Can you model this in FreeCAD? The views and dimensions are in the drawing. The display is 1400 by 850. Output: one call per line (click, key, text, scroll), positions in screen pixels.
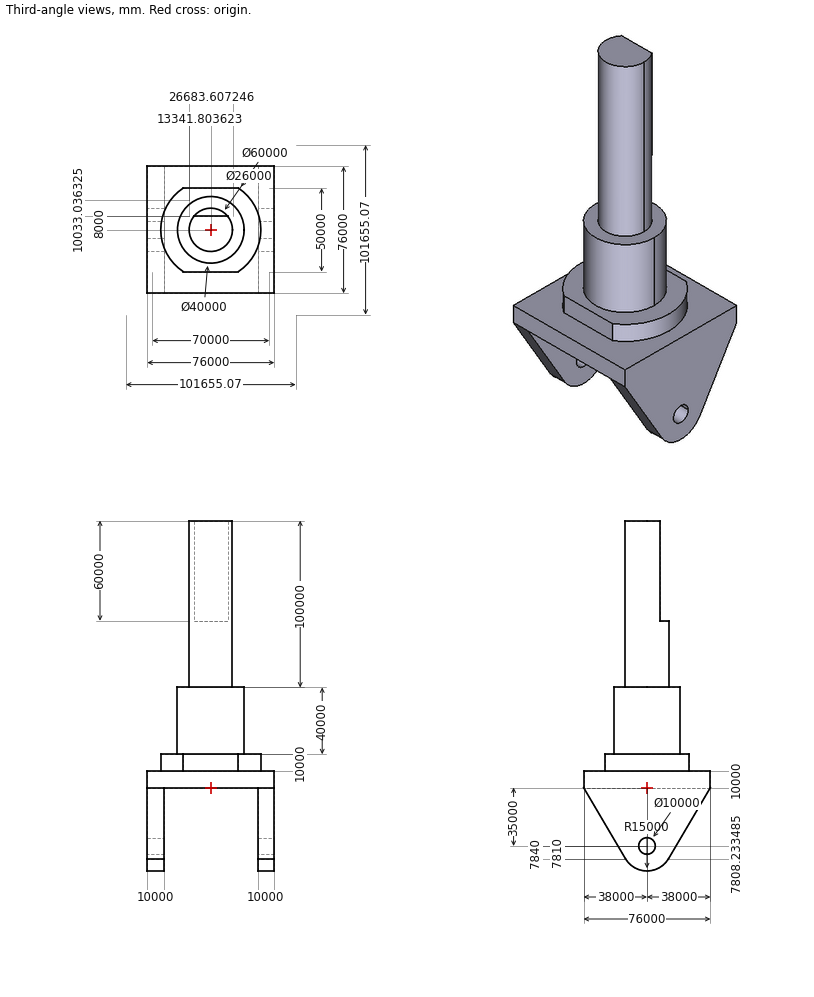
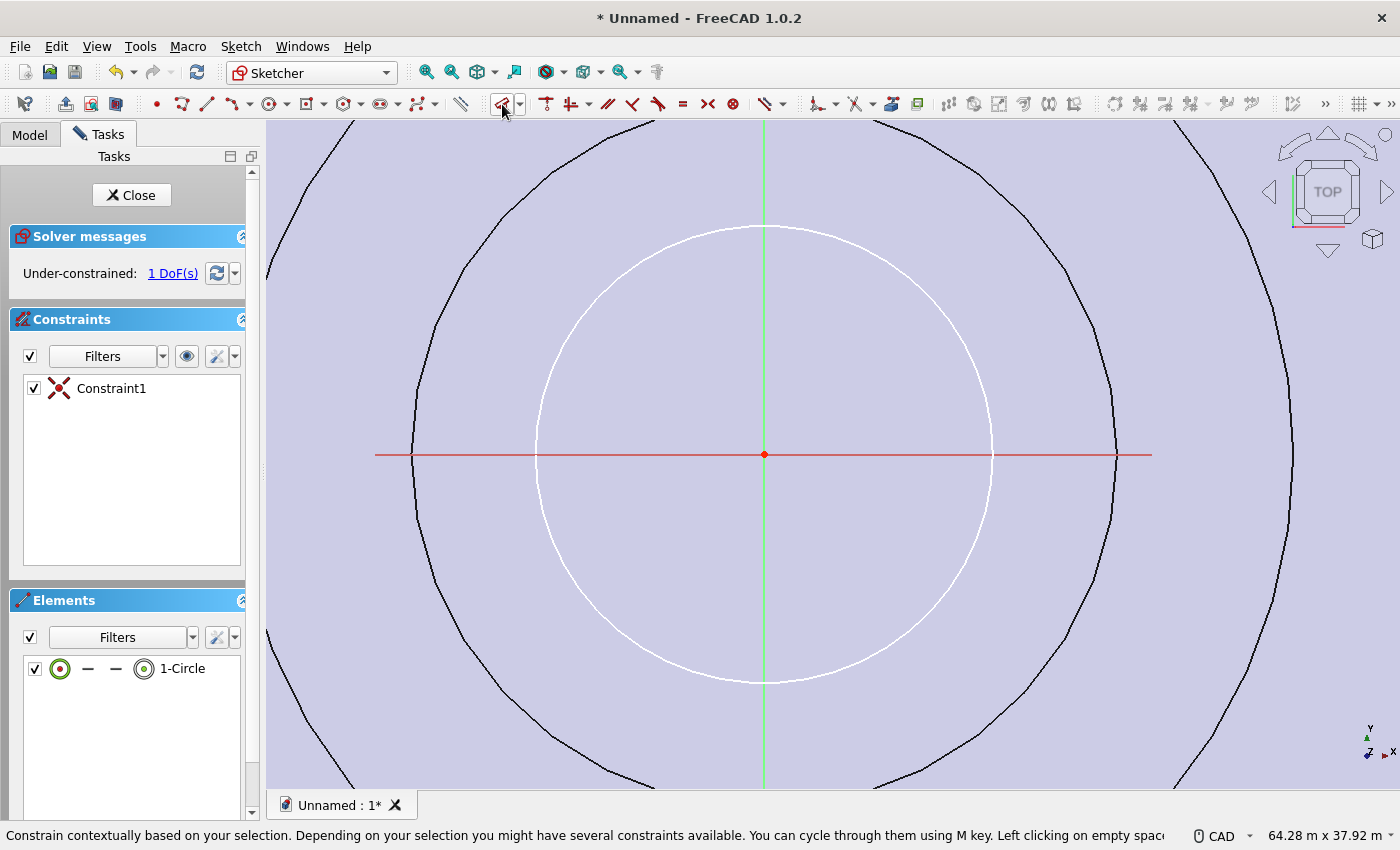
click(925, 292)
click(948, 269)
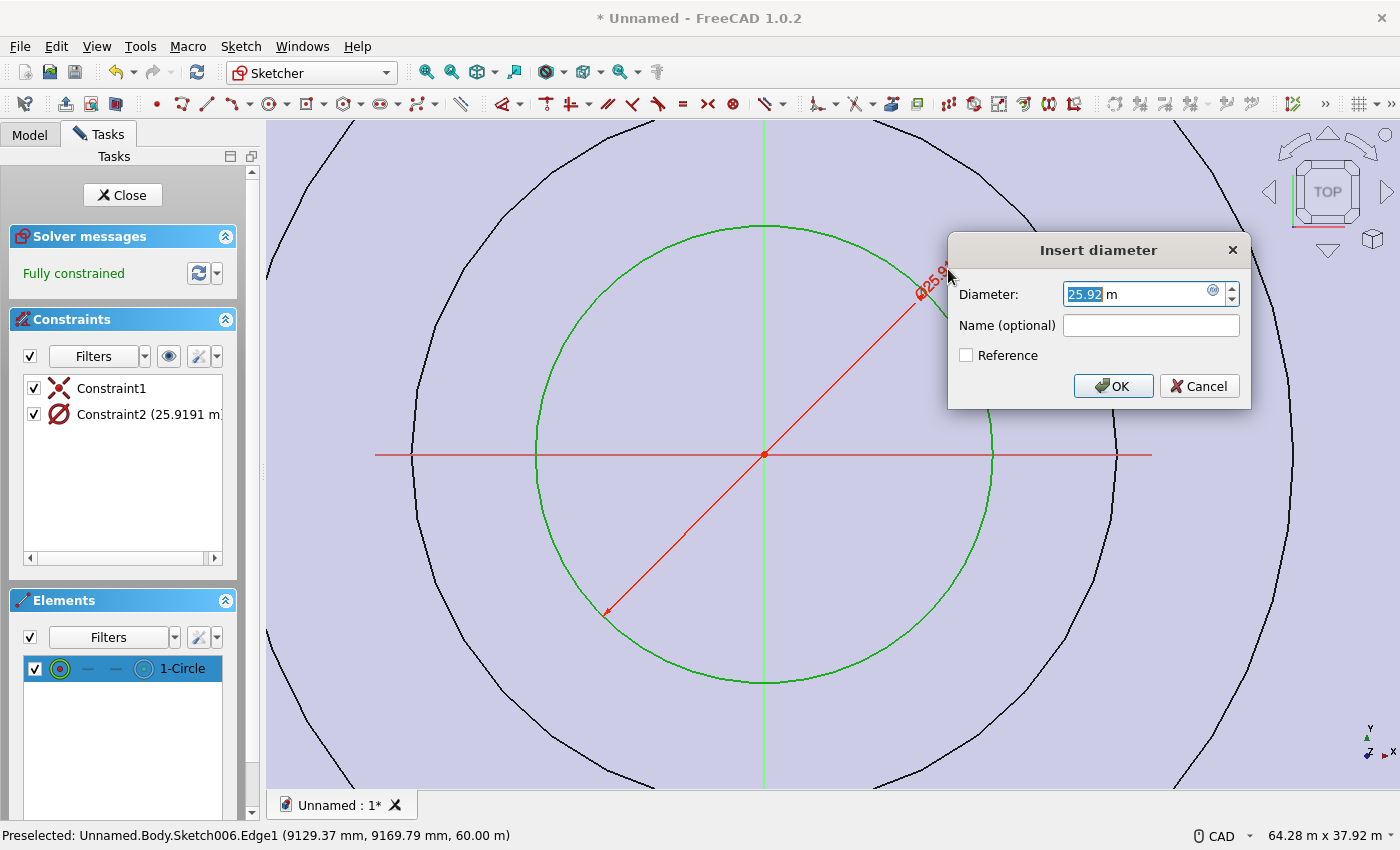
key(ctrl+a)
text(26000 mm)
key(Return)
key(Escape)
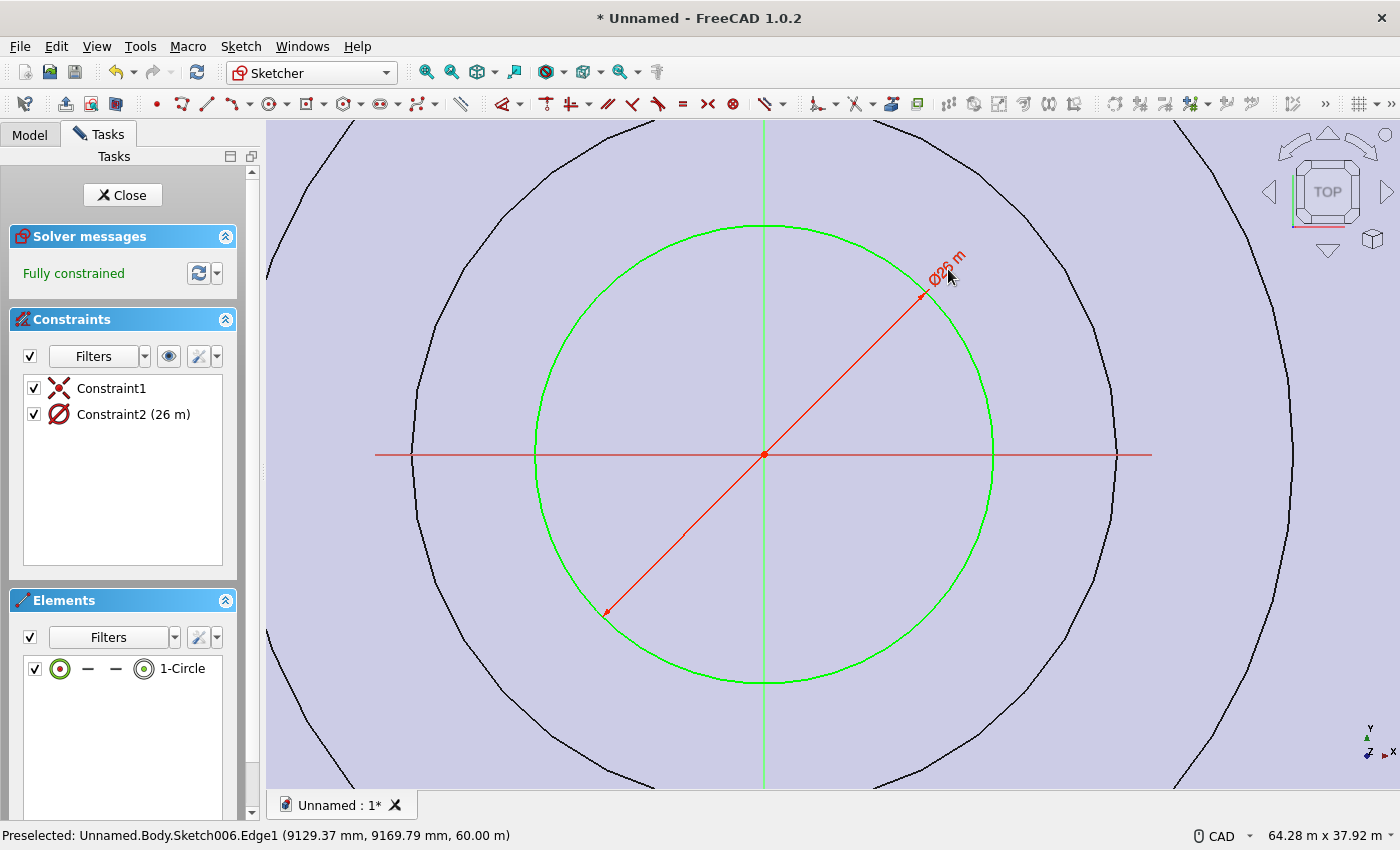
click(123, 195)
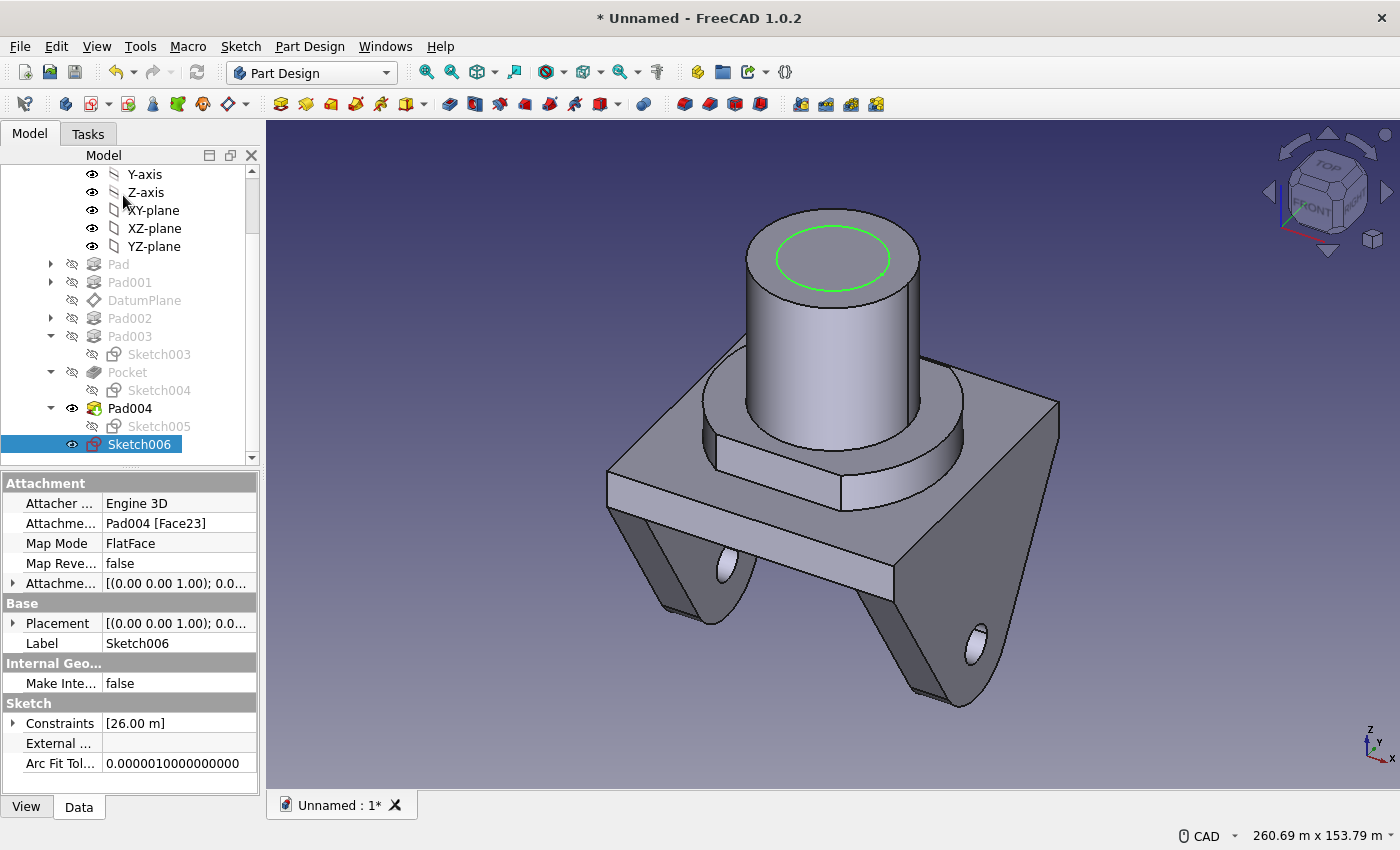
click(281, 104)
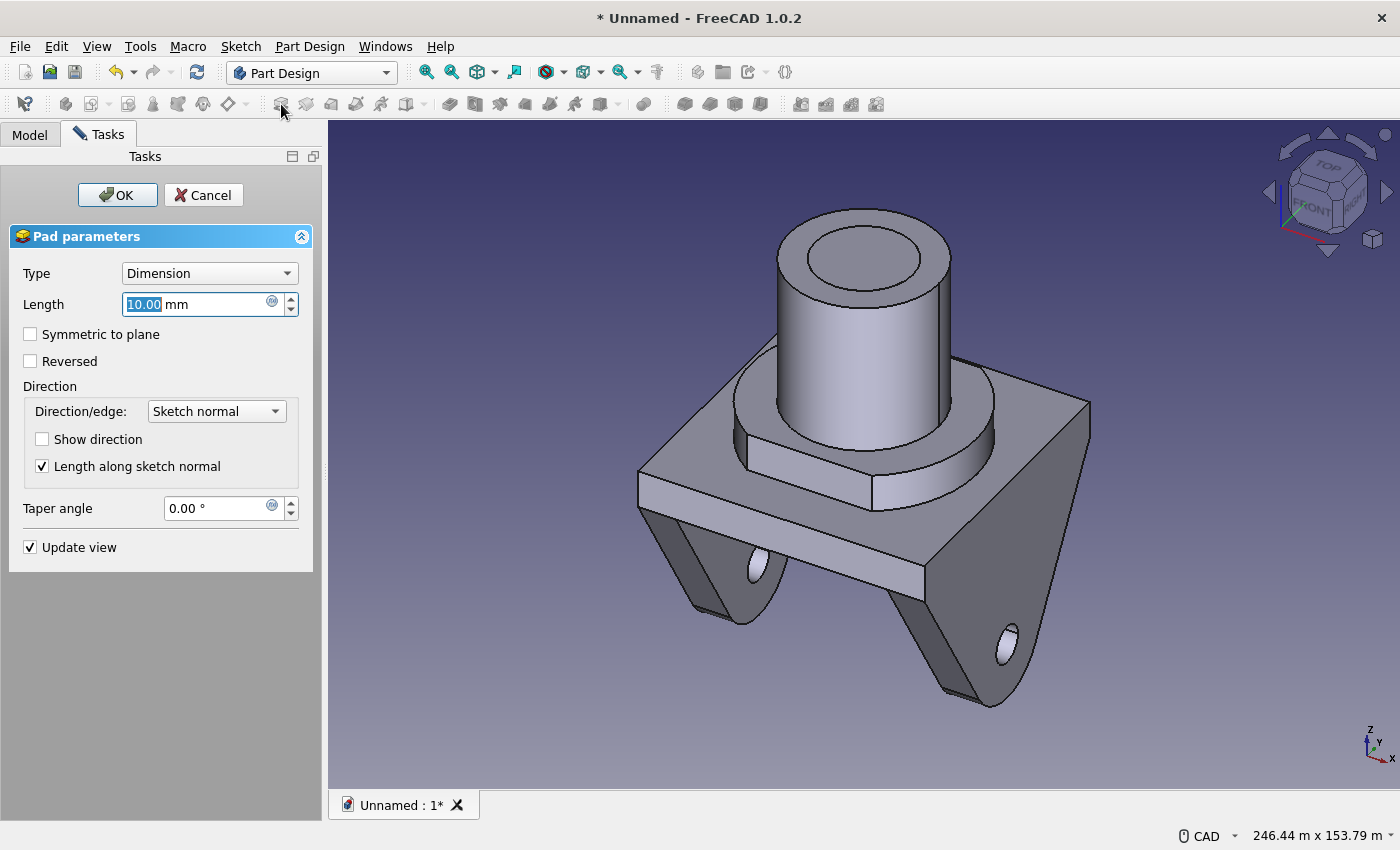
text(100000)
key(Tab)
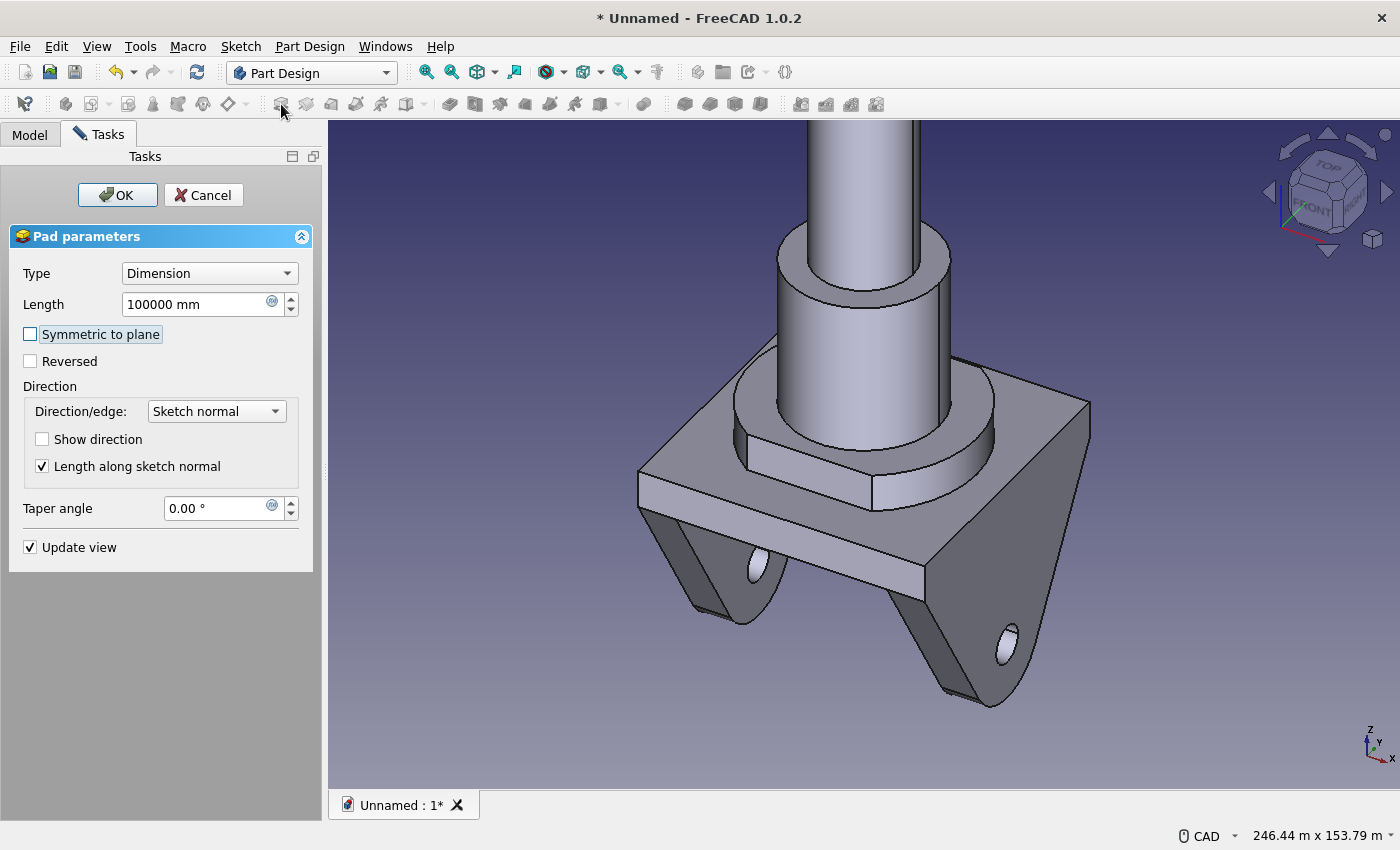
click(118, 195)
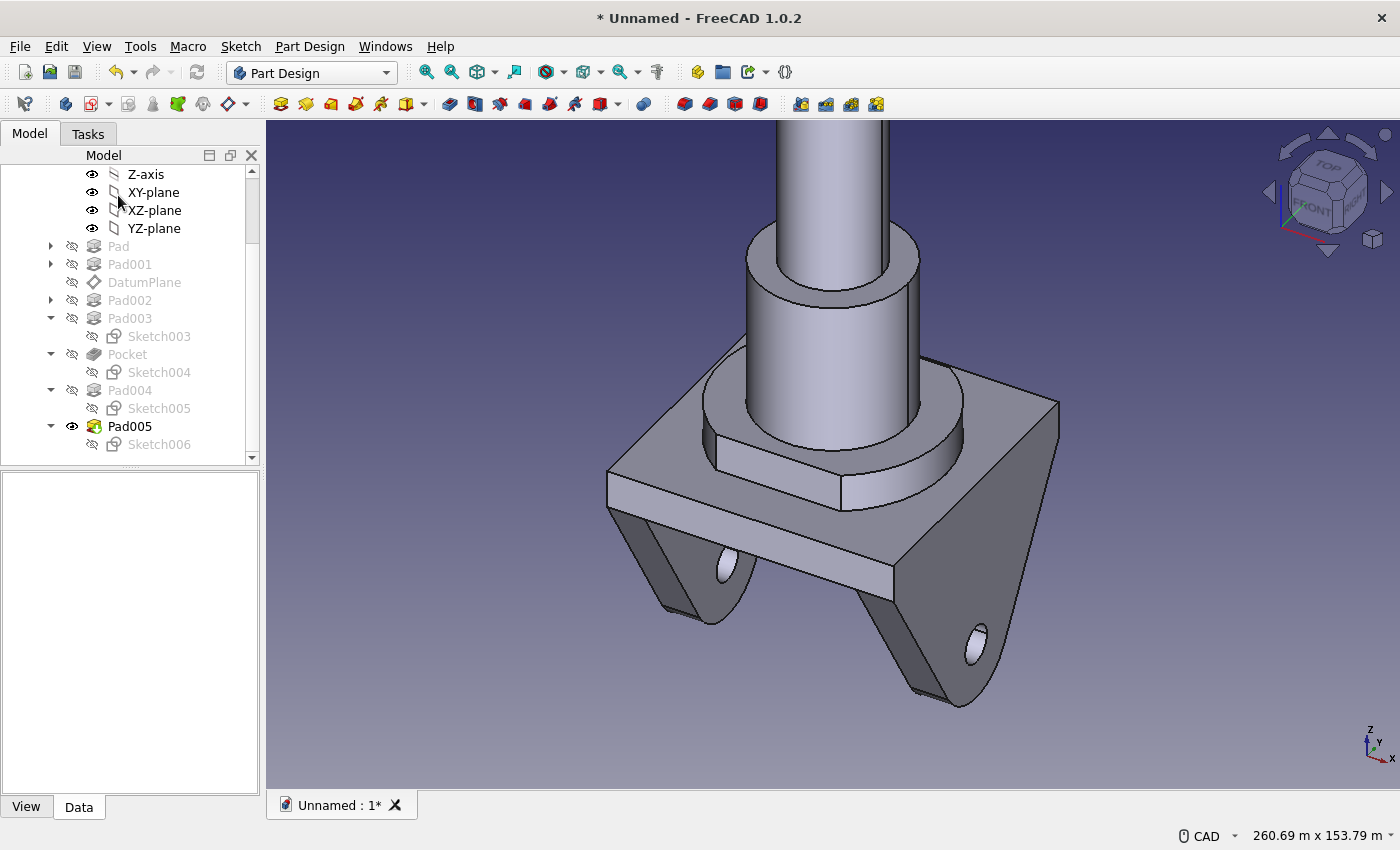
click(427, 72)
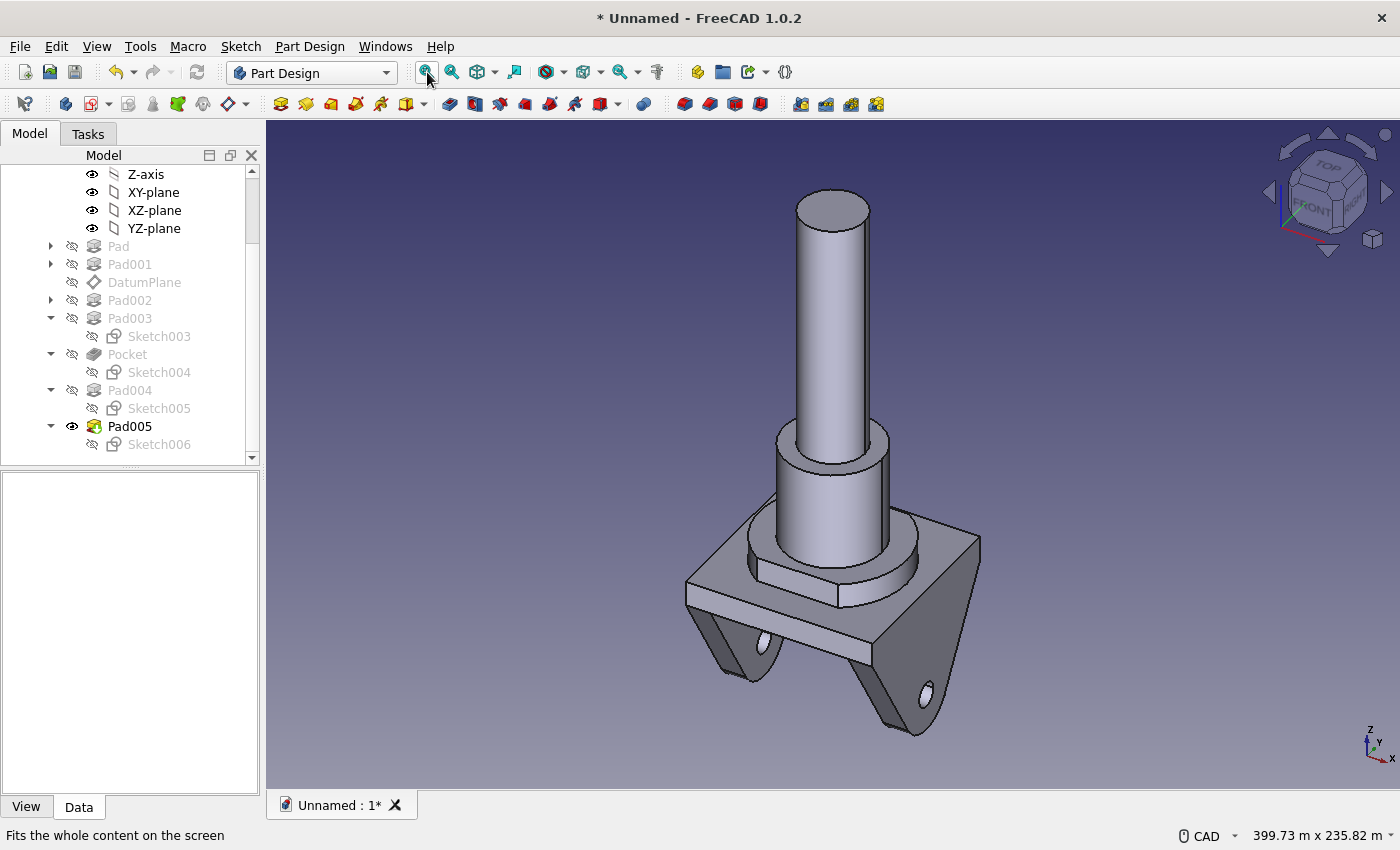
click(833, 210)